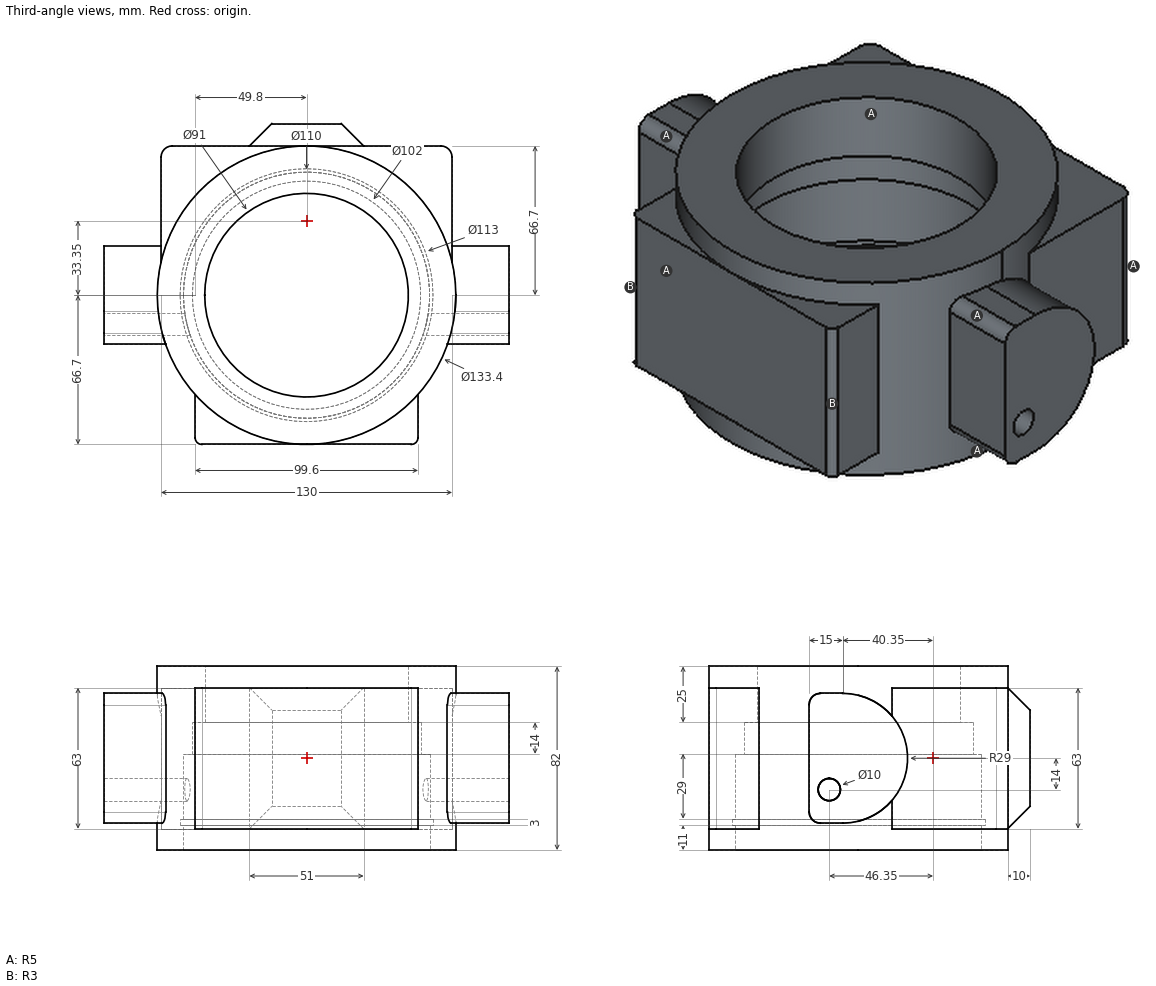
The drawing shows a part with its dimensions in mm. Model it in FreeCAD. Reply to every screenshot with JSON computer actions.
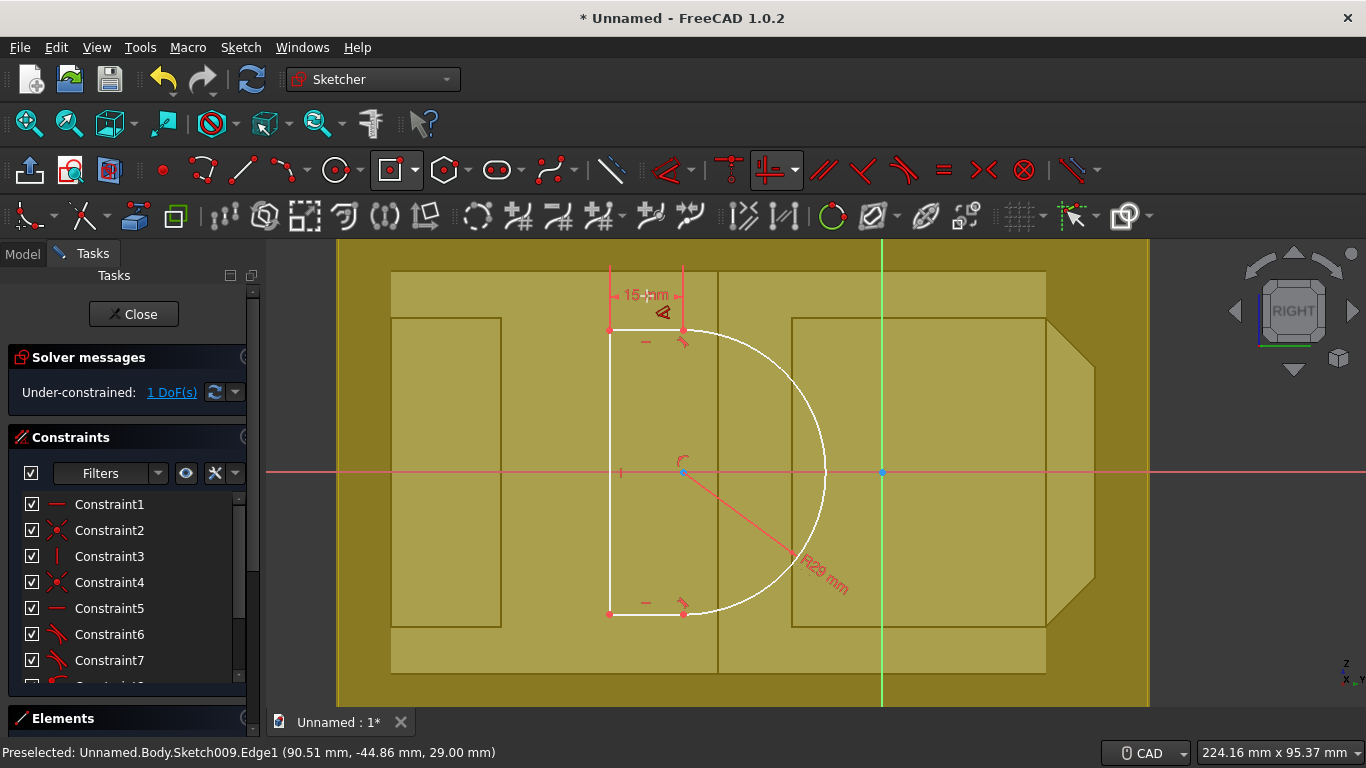
{"action": "left_click", "coordinate": [683, 330]}
{"action": "left_click", "coordinate": [783, 296]}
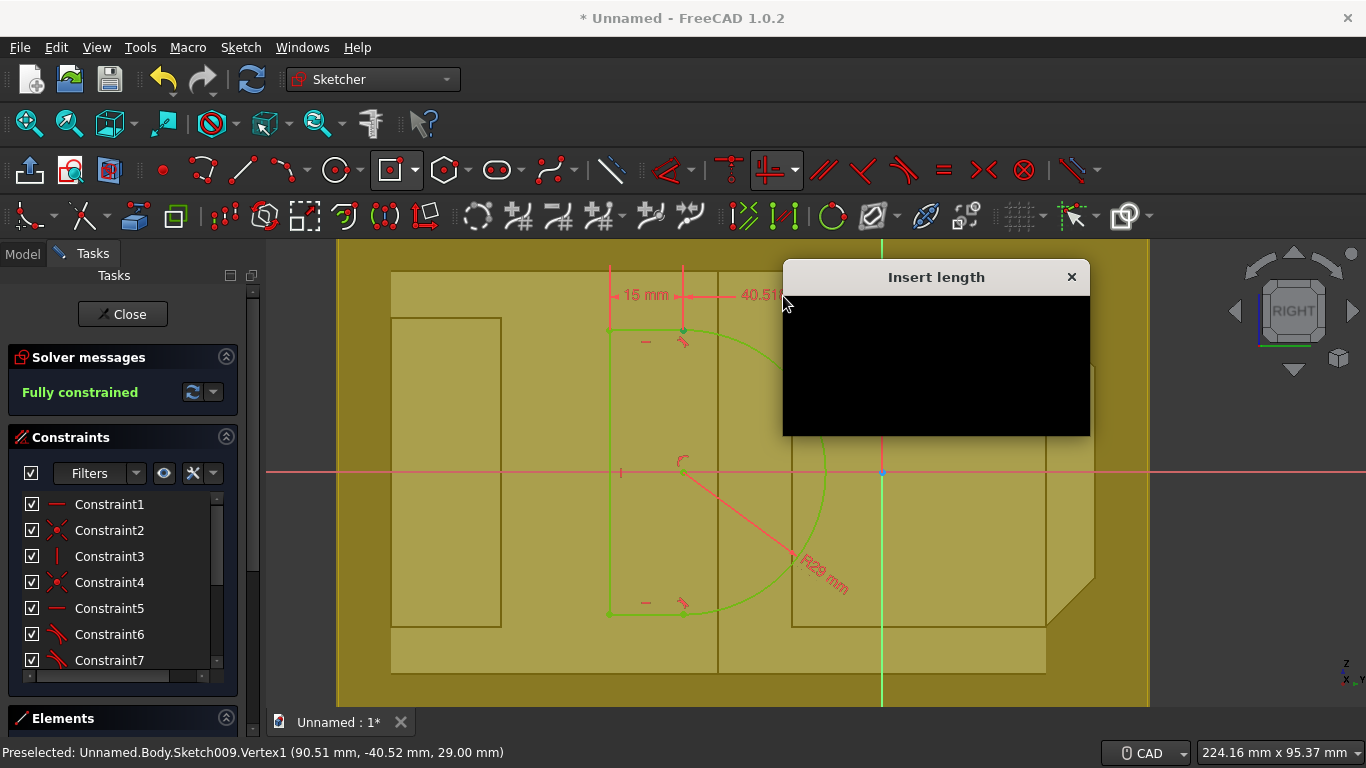
{"action": "type", "text": "40.35"}
{"action": "key", "text": "Return"}
{"action": "key", "text": "Escape"}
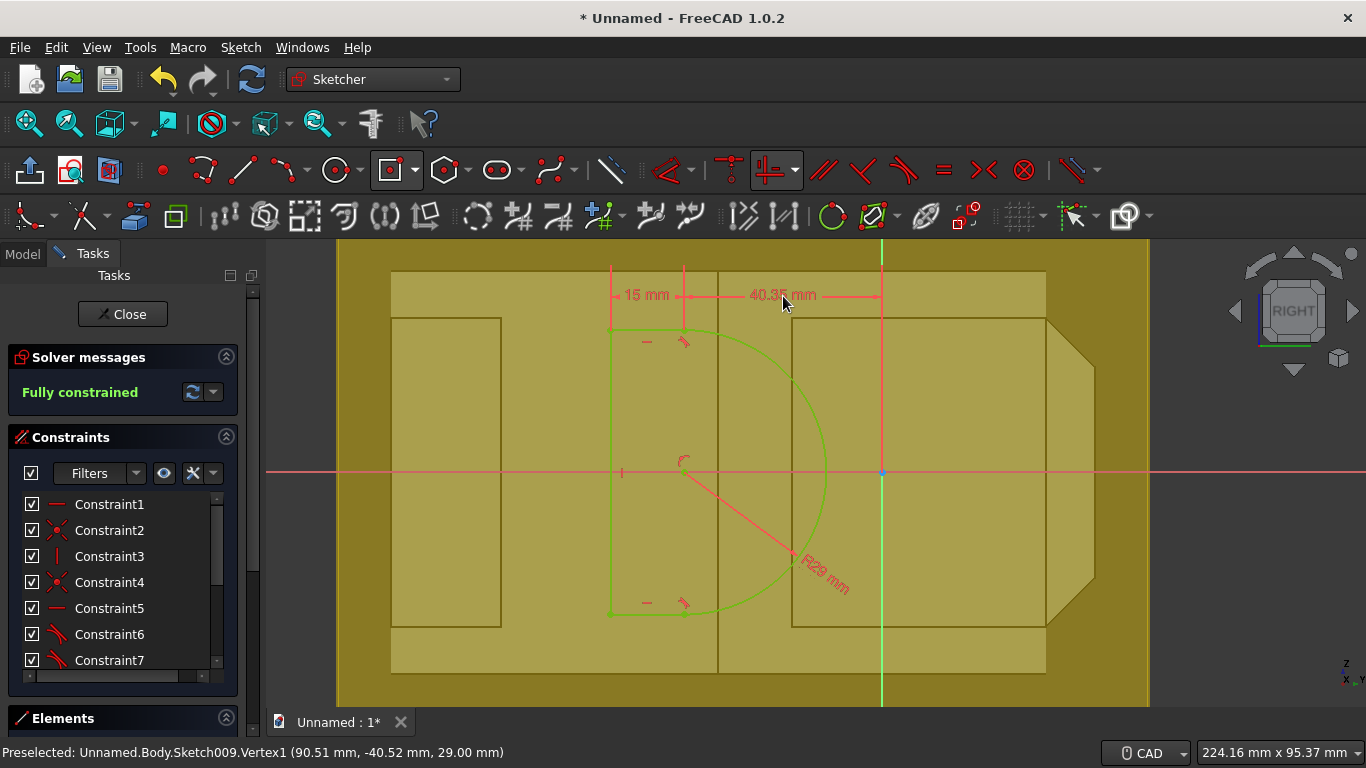
{"action": "left_click", "coordinate": [123, 314]}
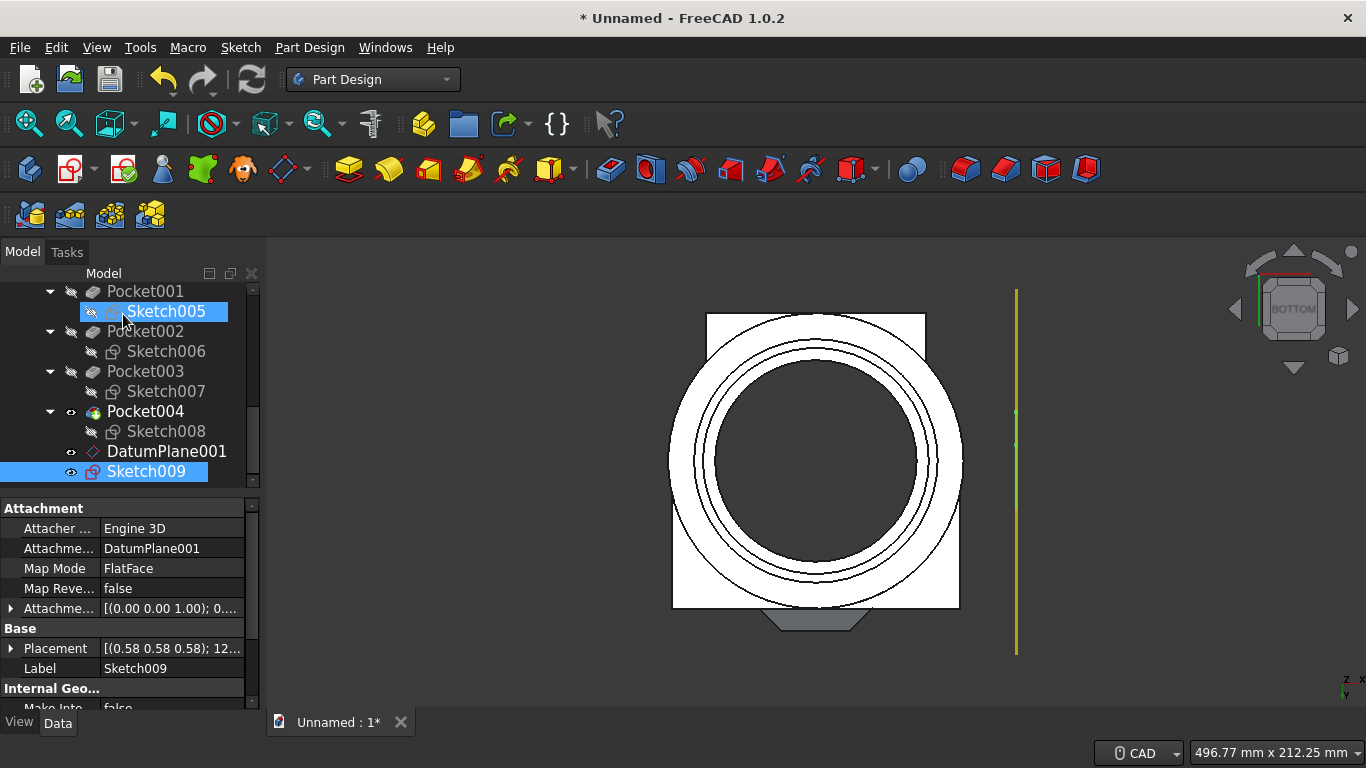
{"action": "left_click", "coordinate": [350, 170]}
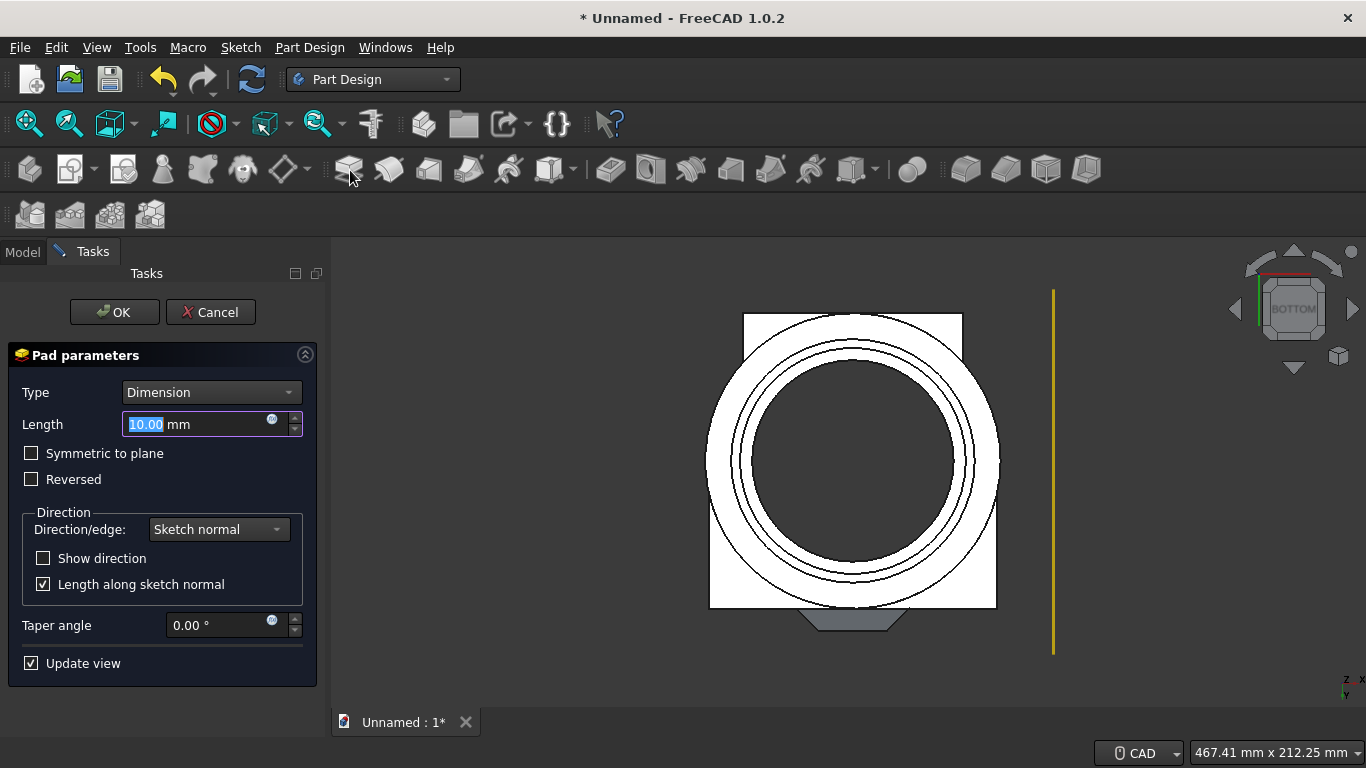
{"action": "left_click", "coordinate": [212, 392]}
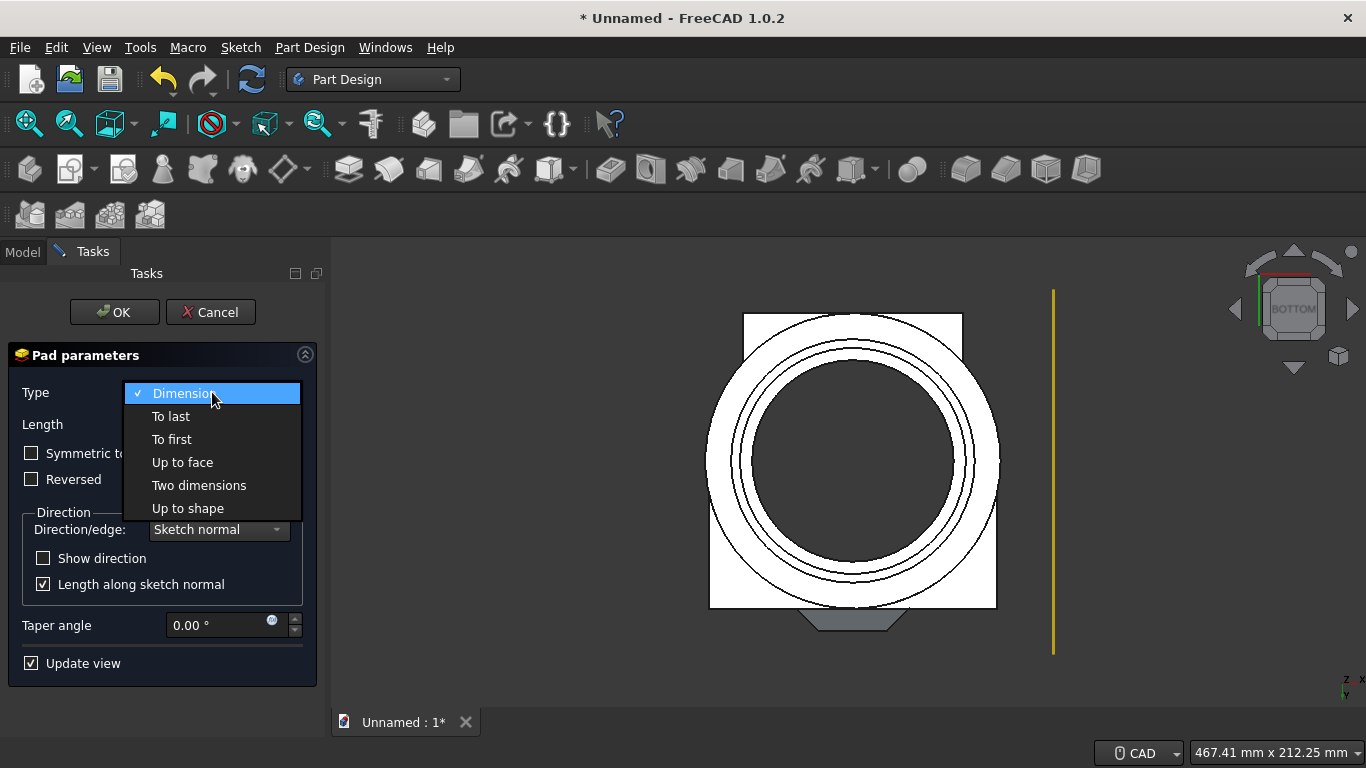
{"action": "left_click", "coordinate": [212, 440]}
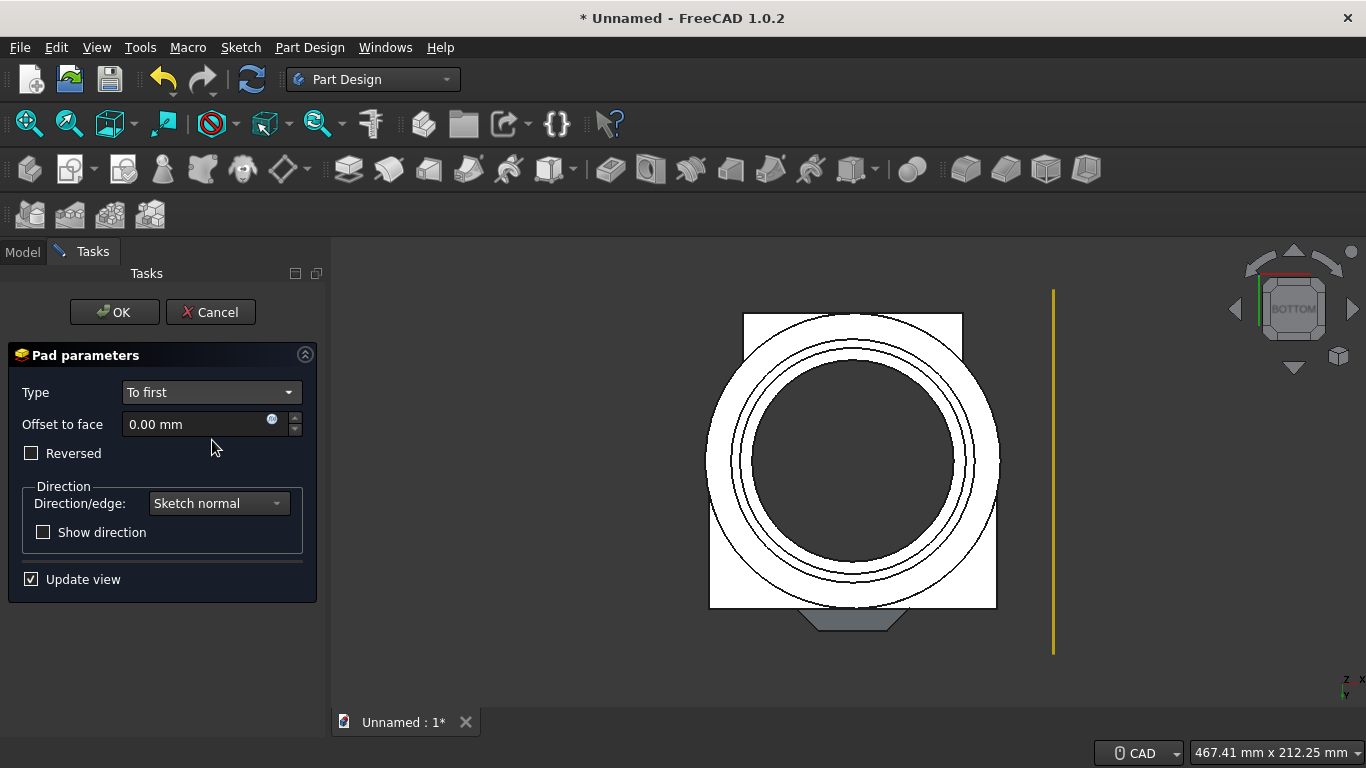
{"action": "left_click", "coordinate": [30, 453]}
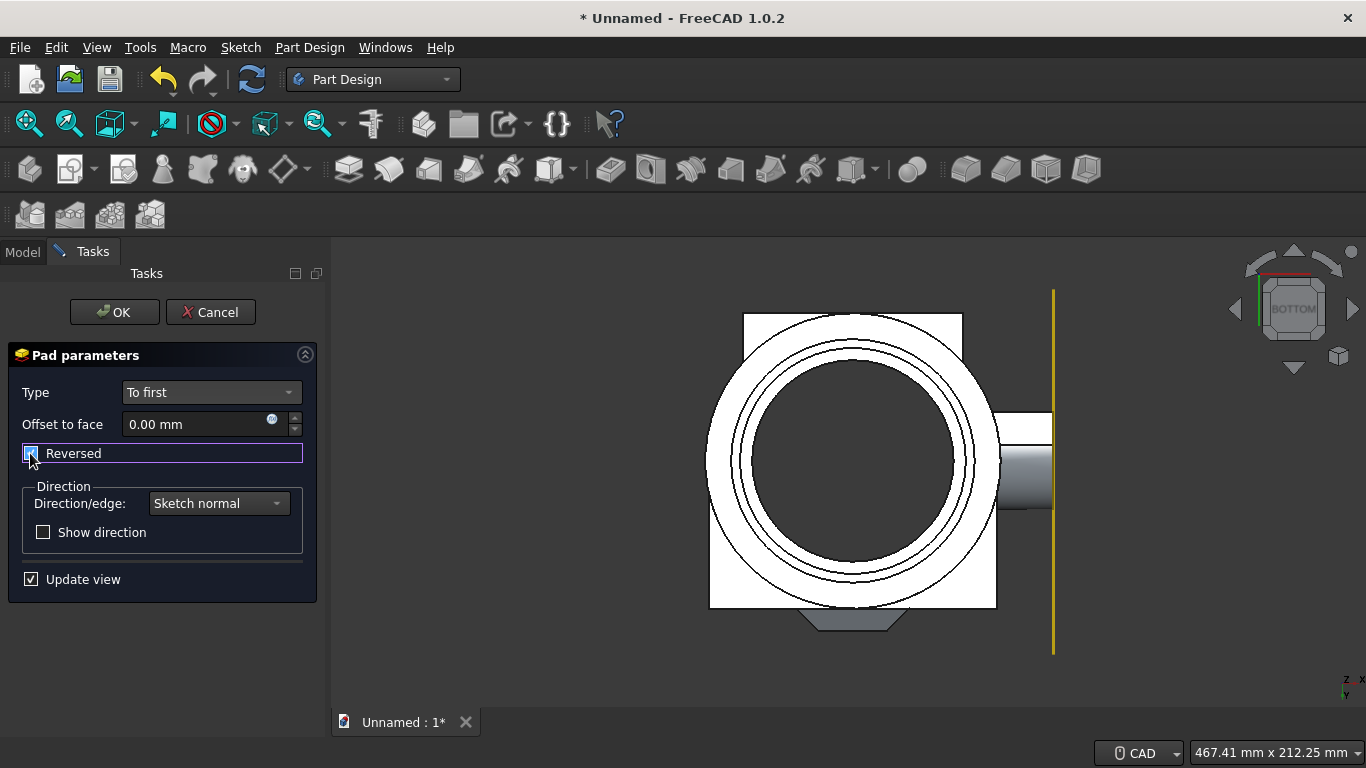
{"action": "left_click", "coordinate": [115, 312]}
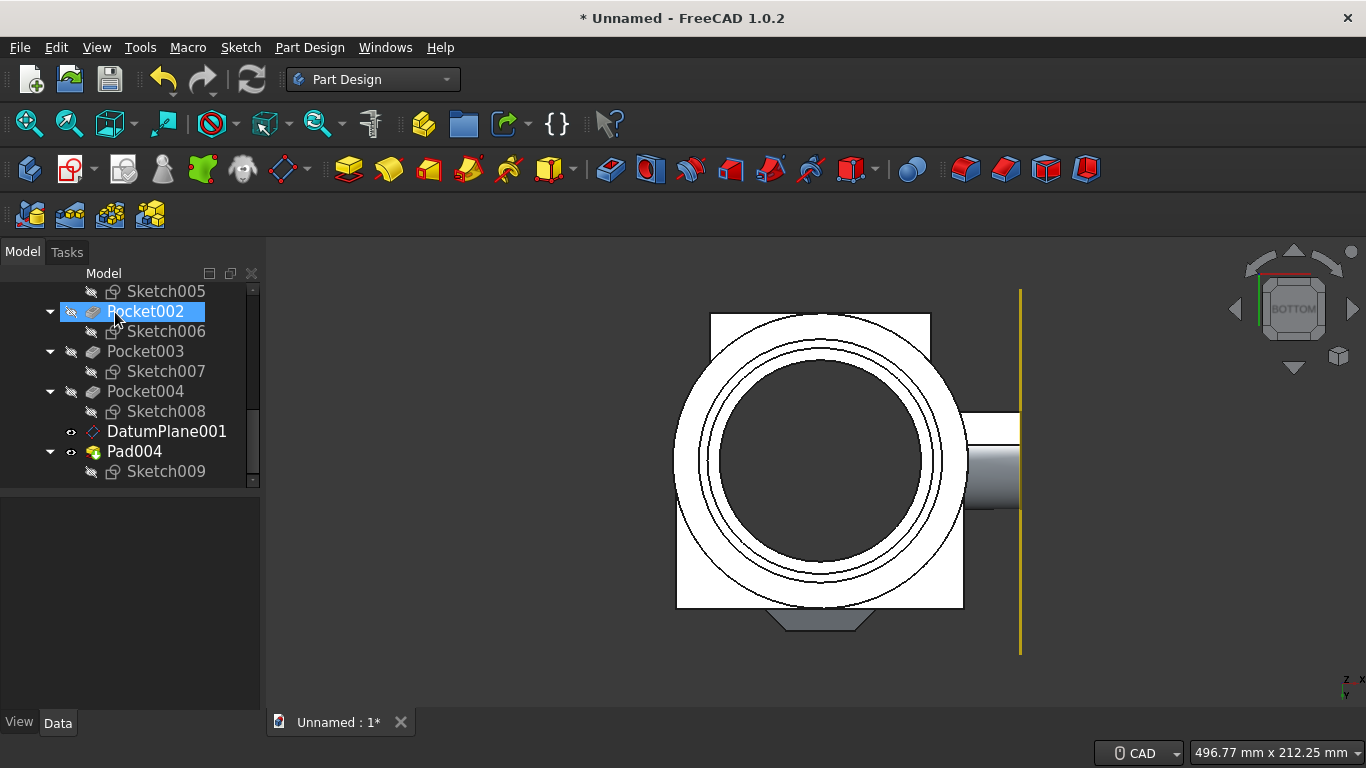
{"action": "left_click", "coordinate": [116, 432]}
{"action": "key", "text": "space"}